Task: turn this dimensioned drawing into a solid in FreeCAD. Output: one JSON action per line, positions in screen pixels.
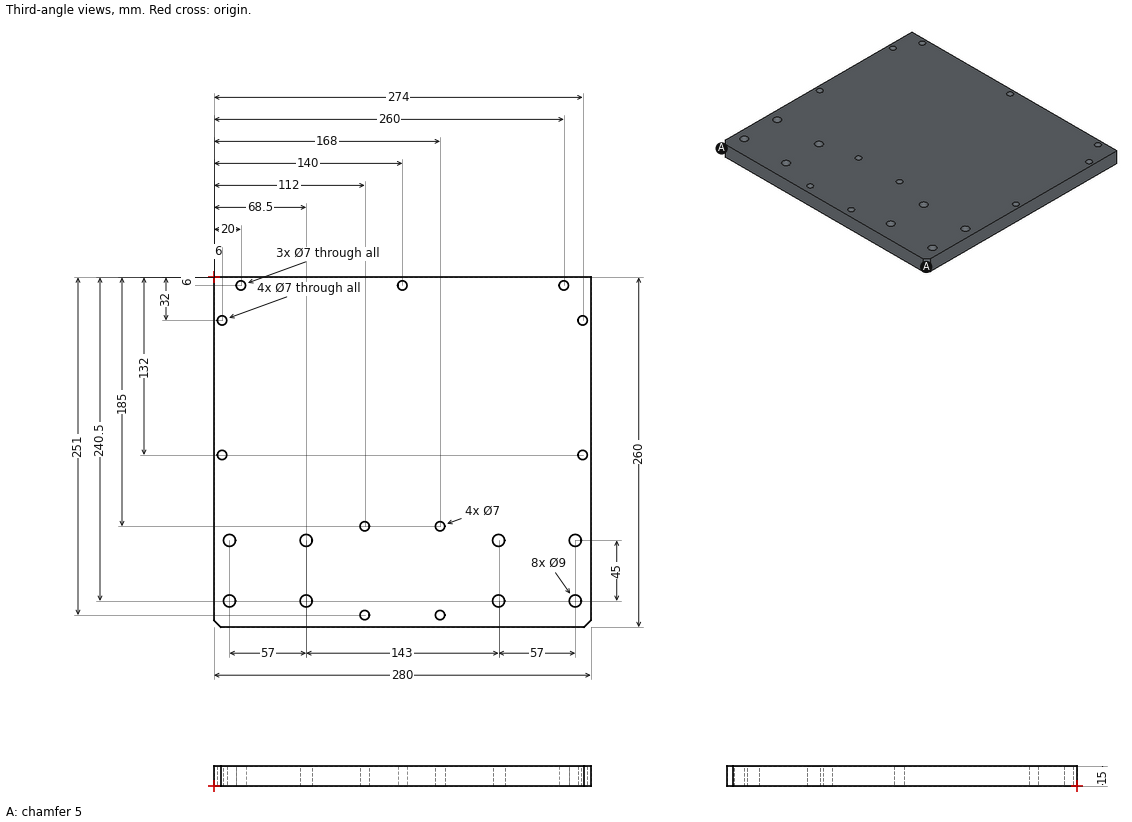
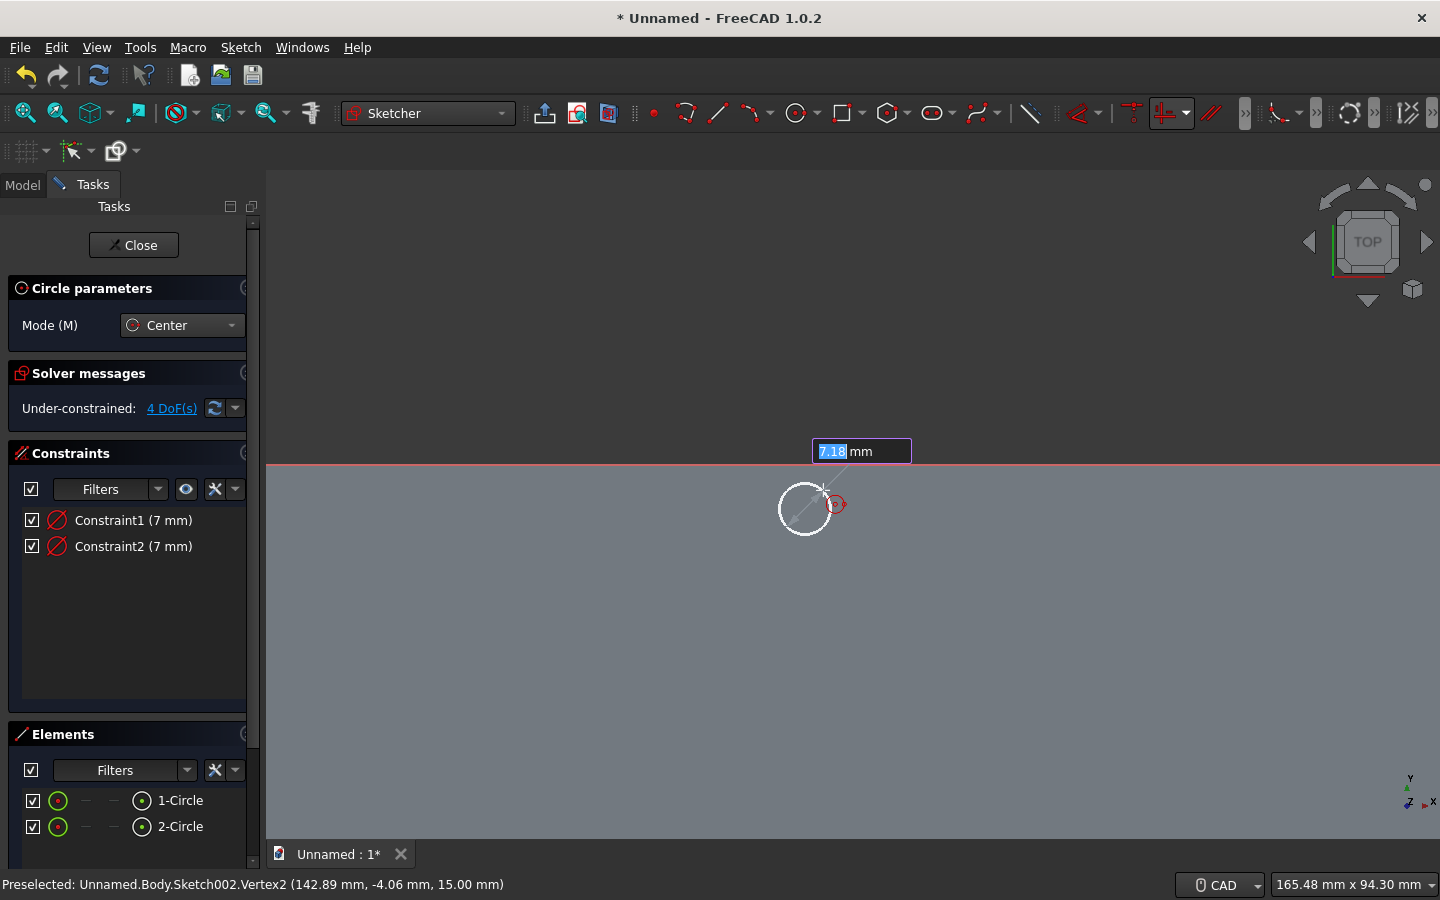
{"action": "type", "text": "7"}
{"action": "key", "text": "Return"}
{"action": "key", "text": "Escape"}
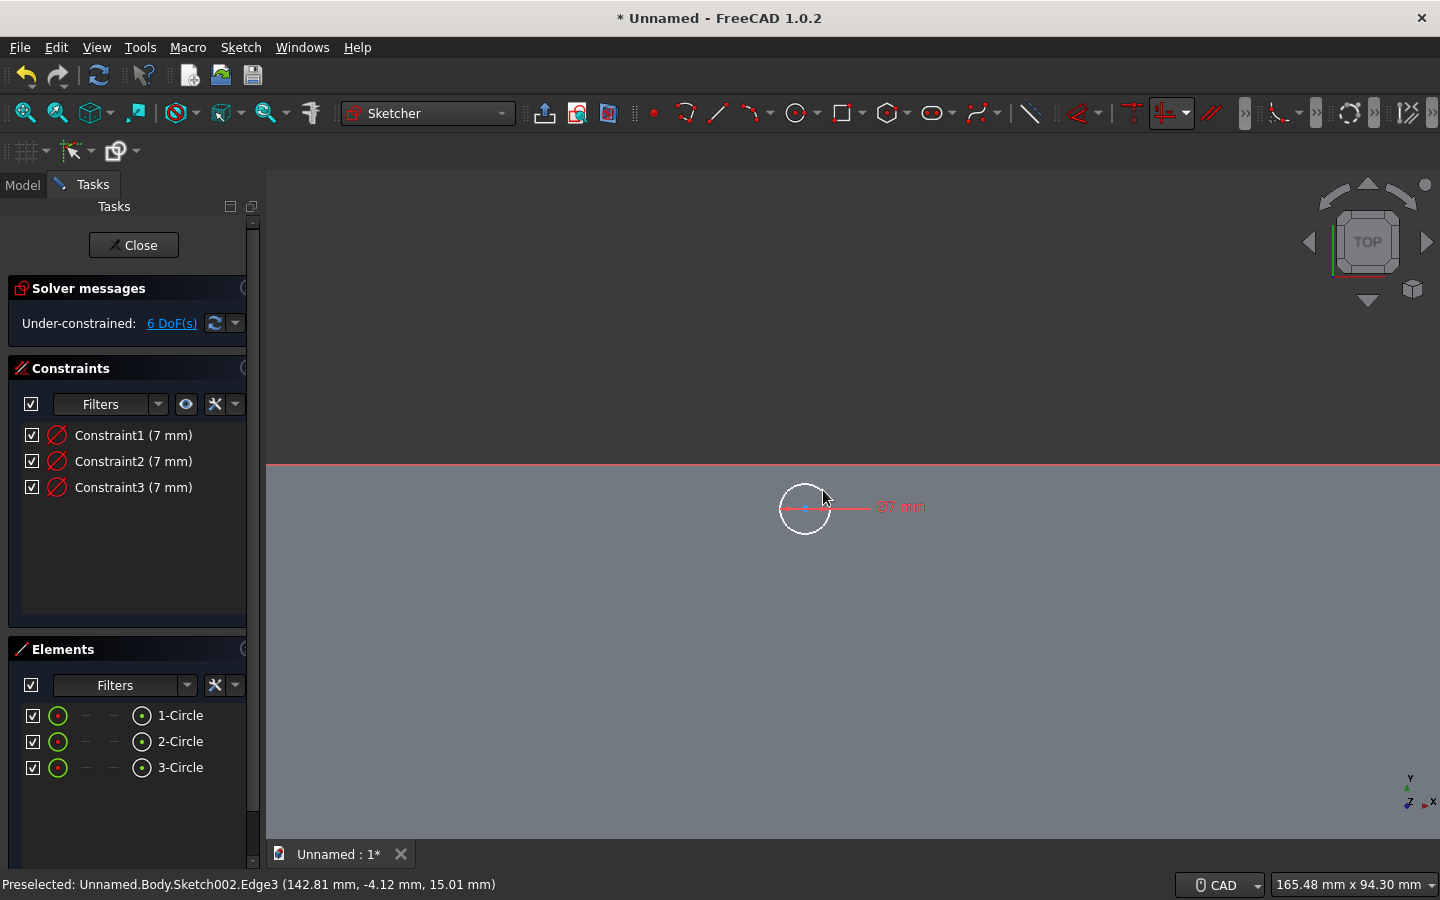
{"action": "scroll", "coordinate": [807, 508], "scroll_direction": "down", "scroll_amount": 5}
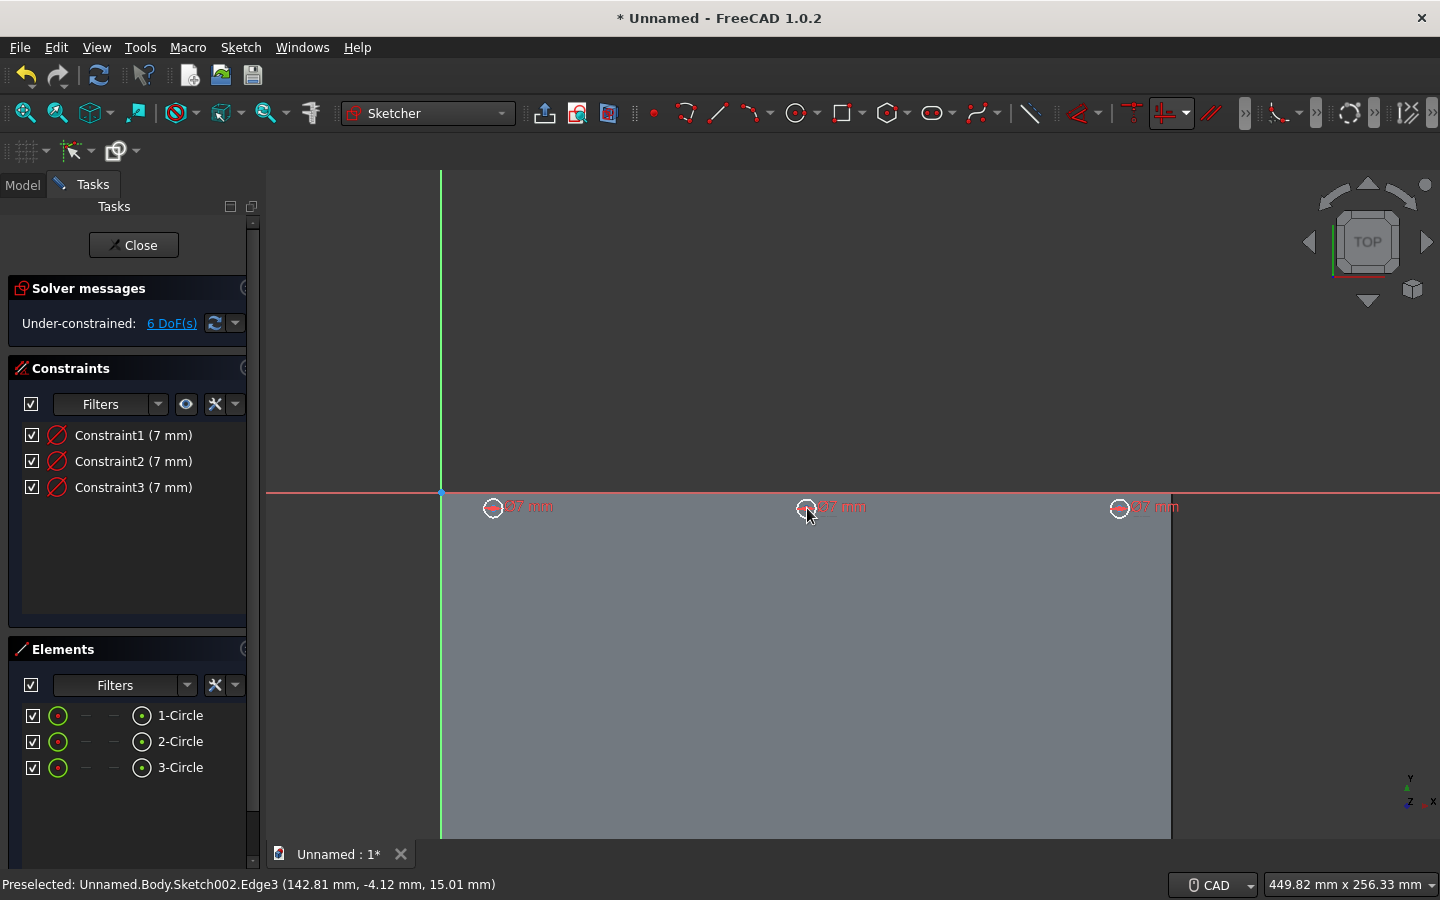
{"action": "left_click", "coordinate": [493, 508]}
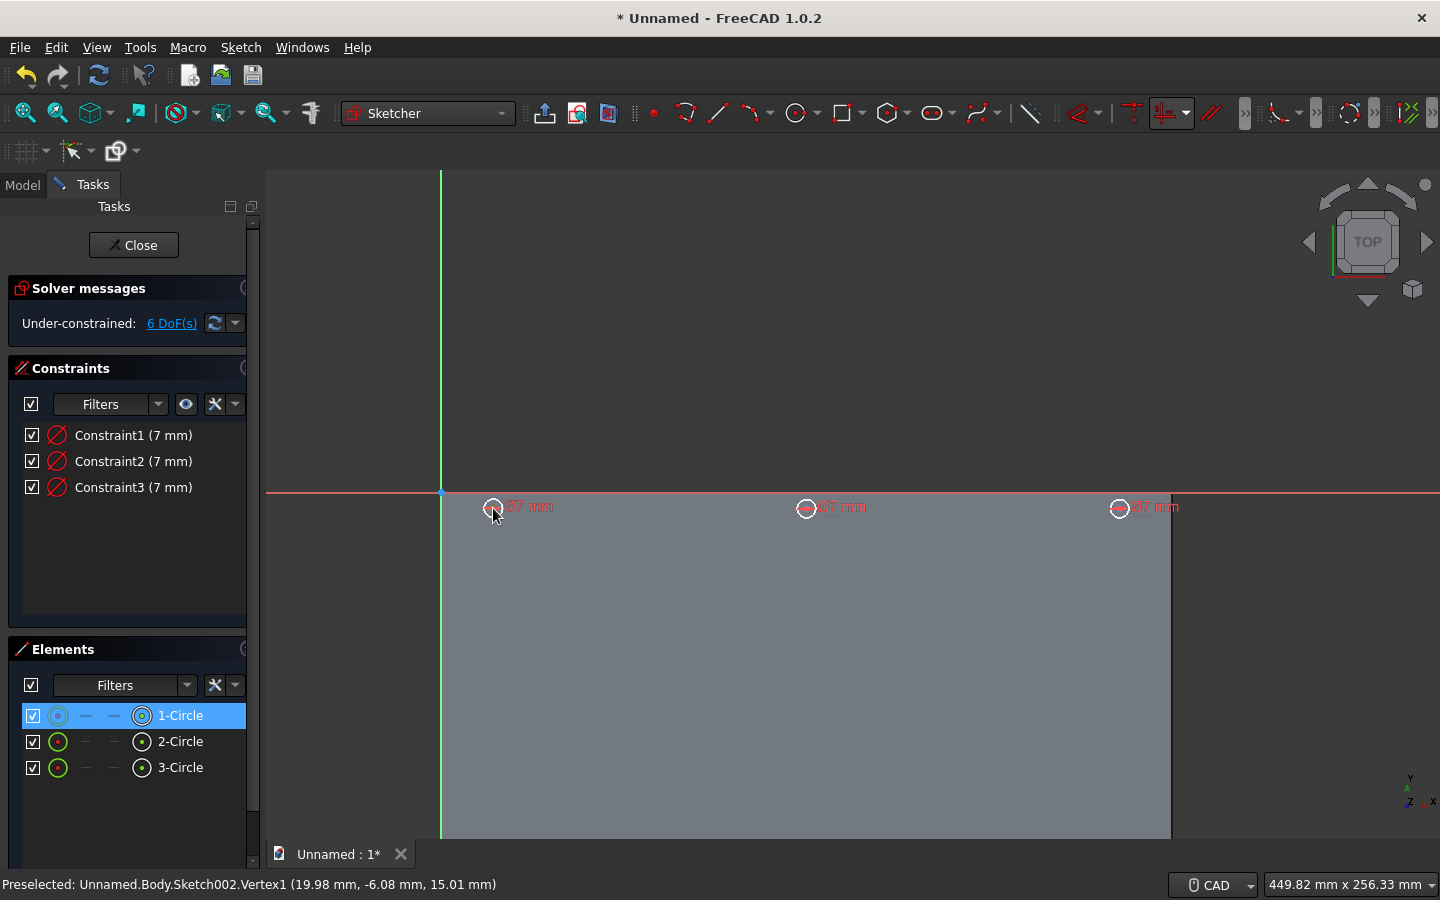
{"action": "left_click", "coordinate": [1120, 509]}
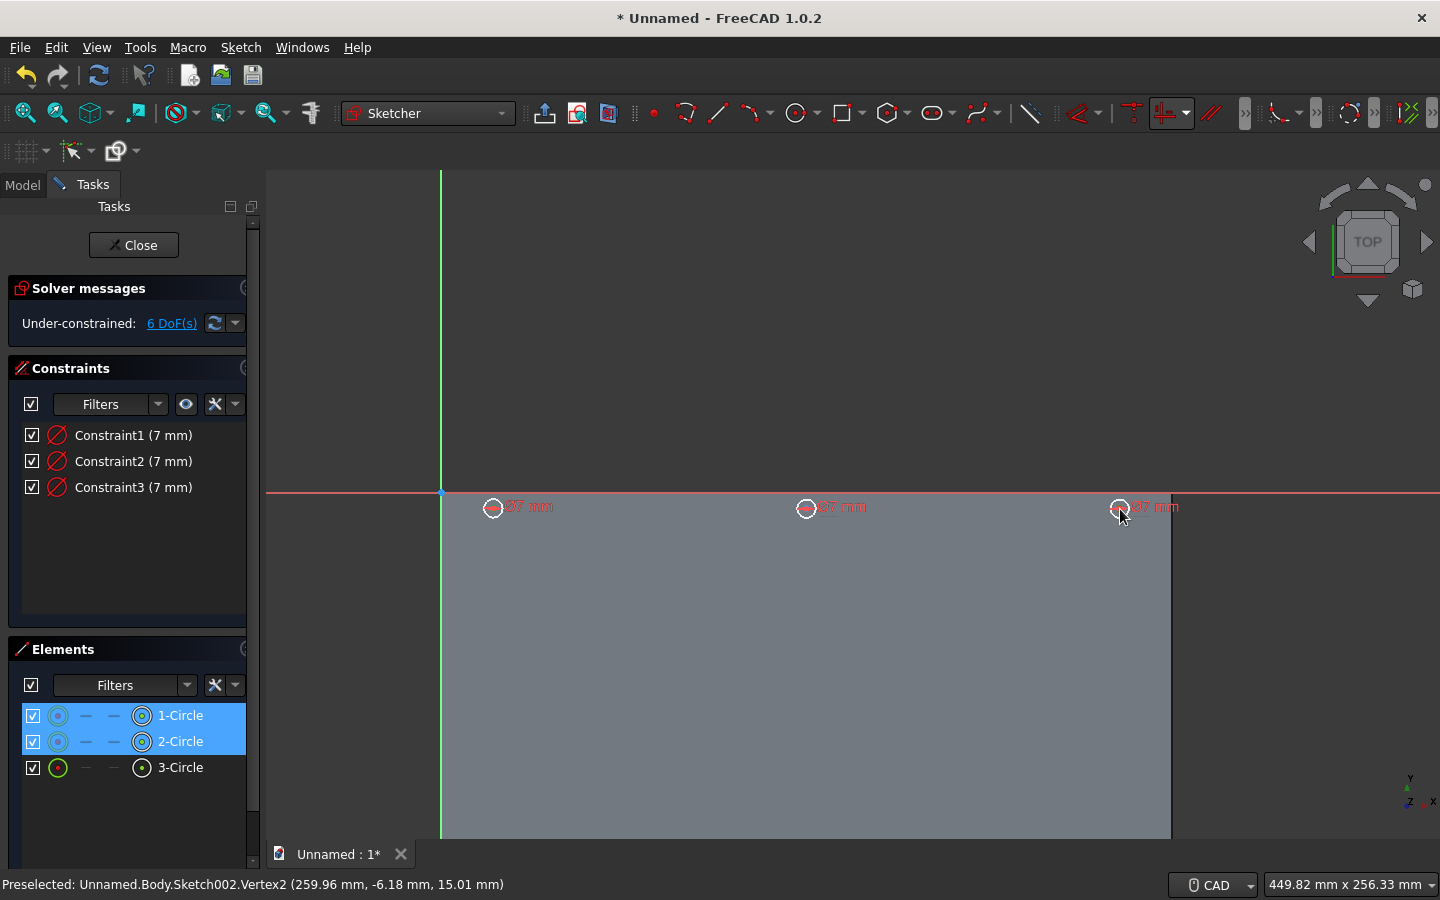
{"action": "left_click", "coordinate": [1188, 114]}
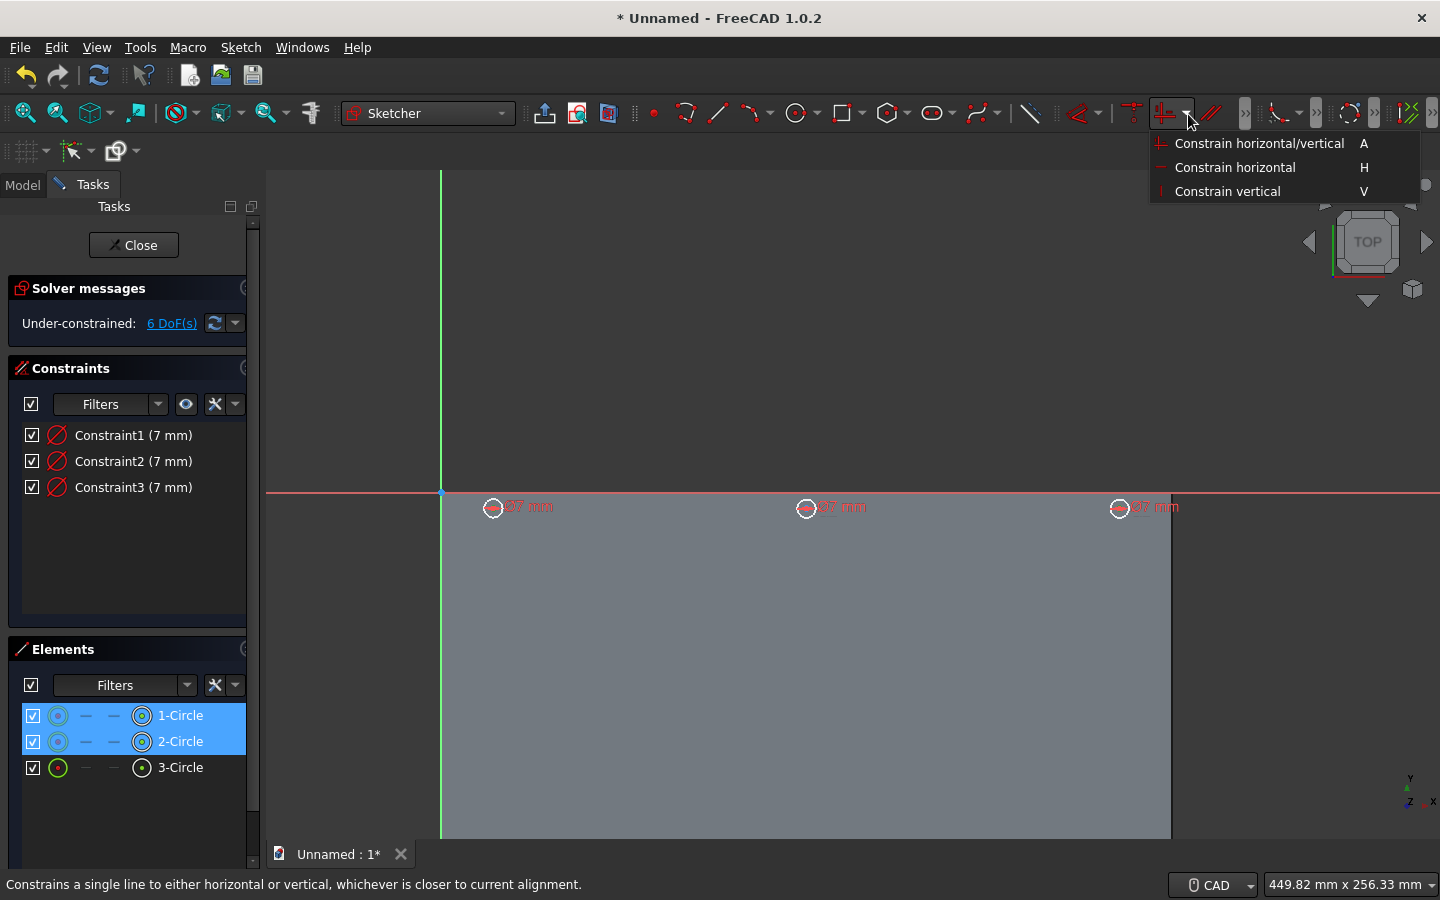
{"action": "left_click", "coordinate": [1285, 167]}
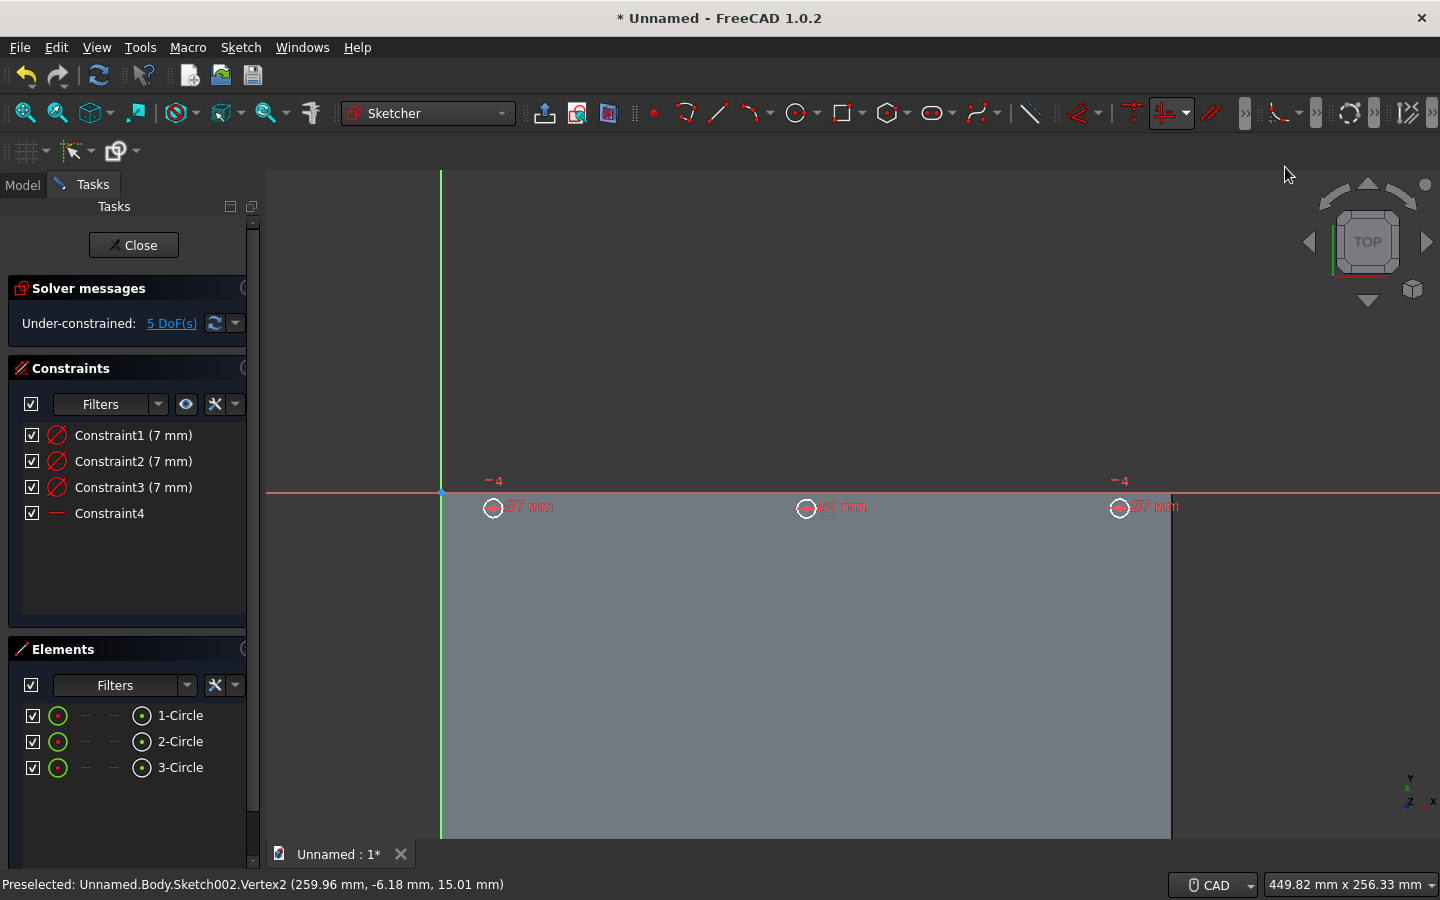
{"action": "left_click", "coordinate": [493, 508]}